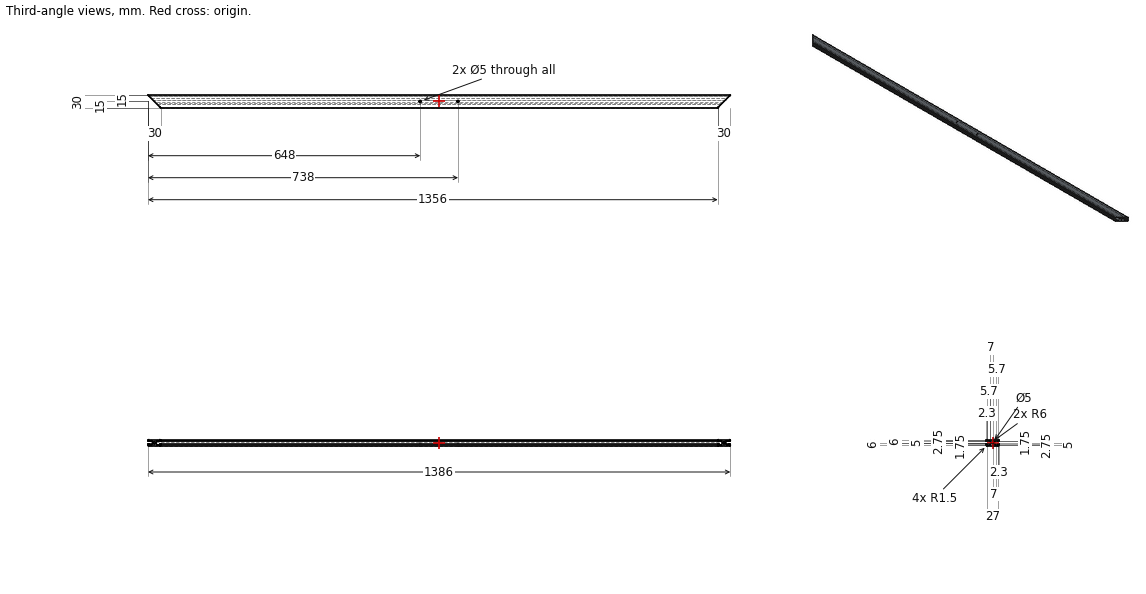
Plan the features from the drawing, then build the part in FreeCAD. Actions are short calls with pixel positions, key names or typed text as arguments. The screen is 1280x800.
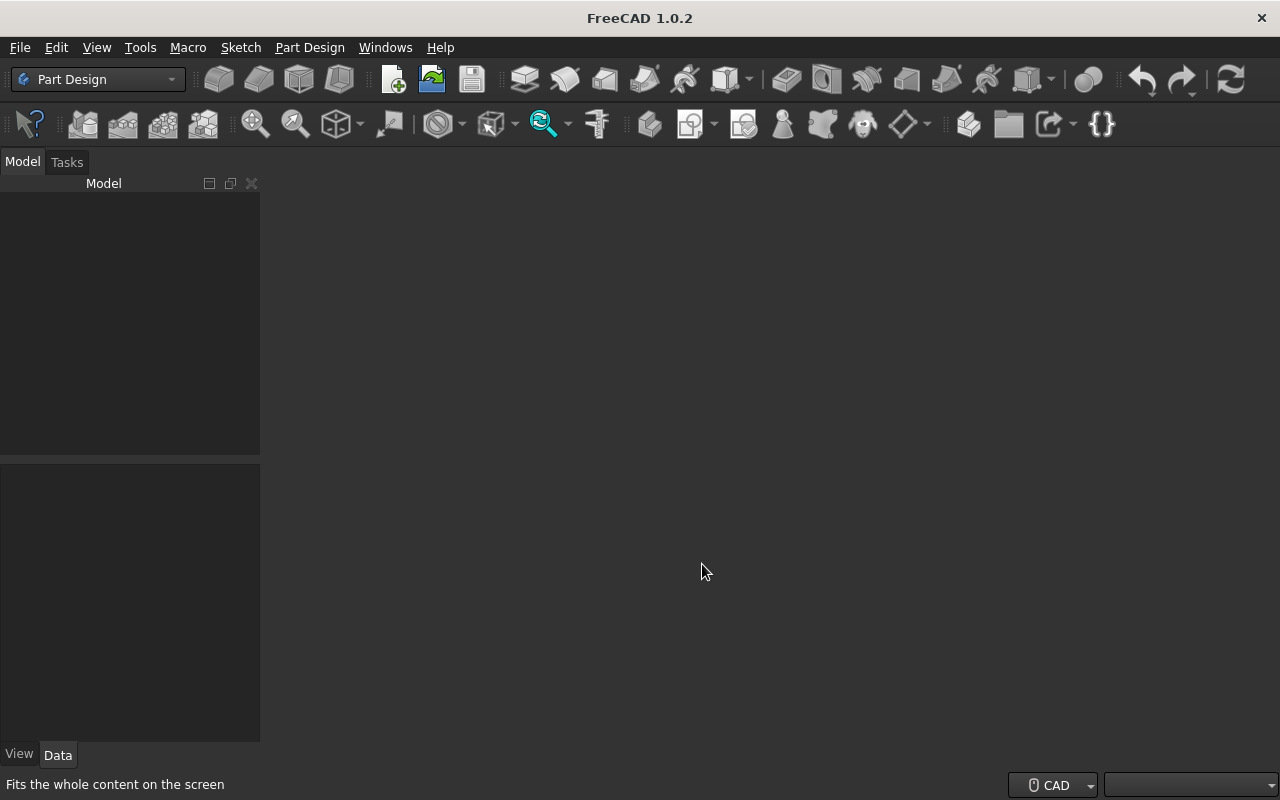
click(392, 80)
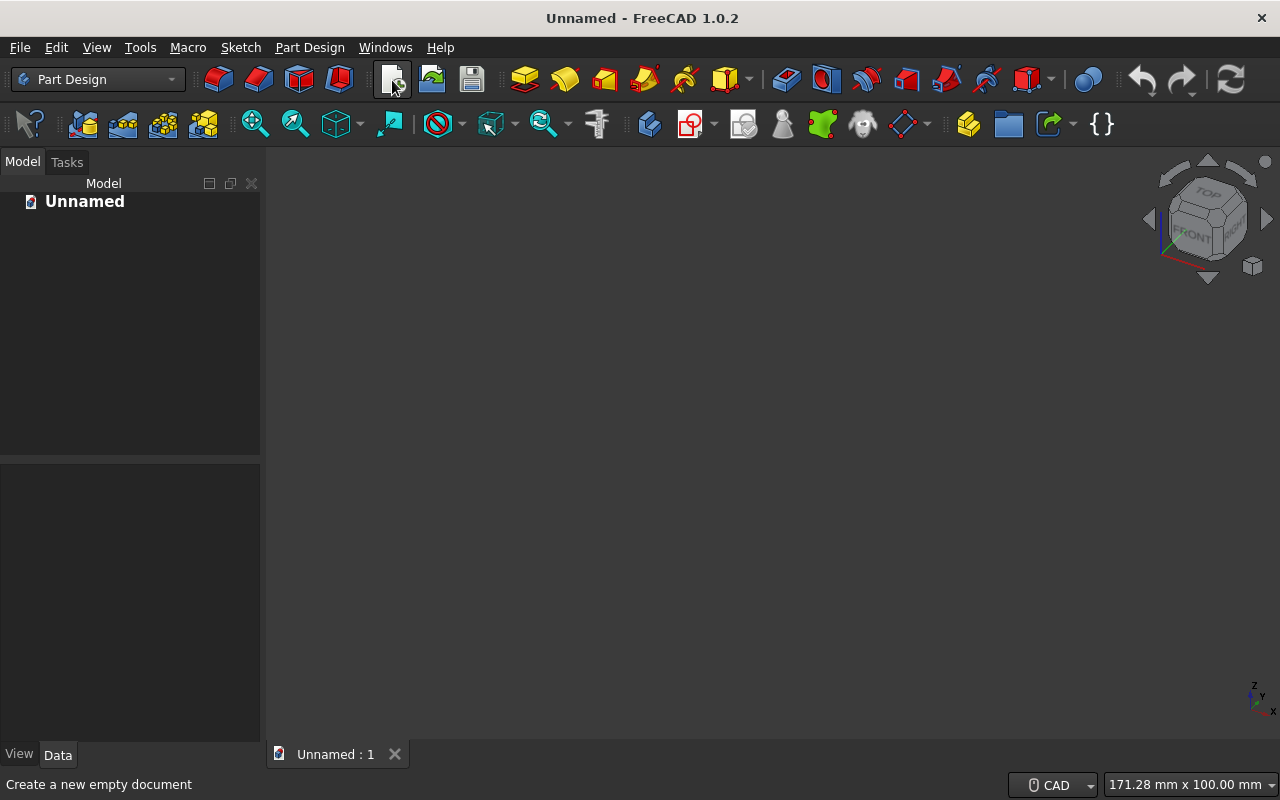
click(650, 124)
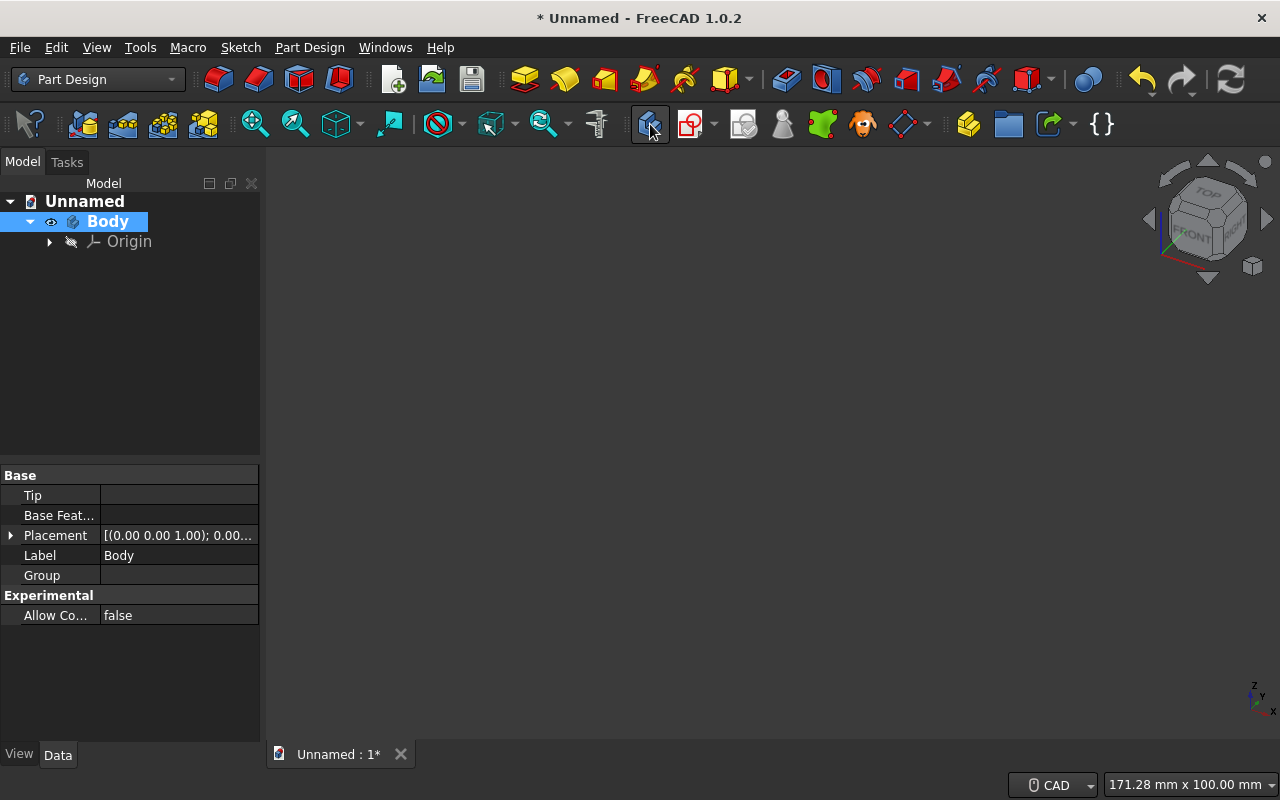
click(50, 242)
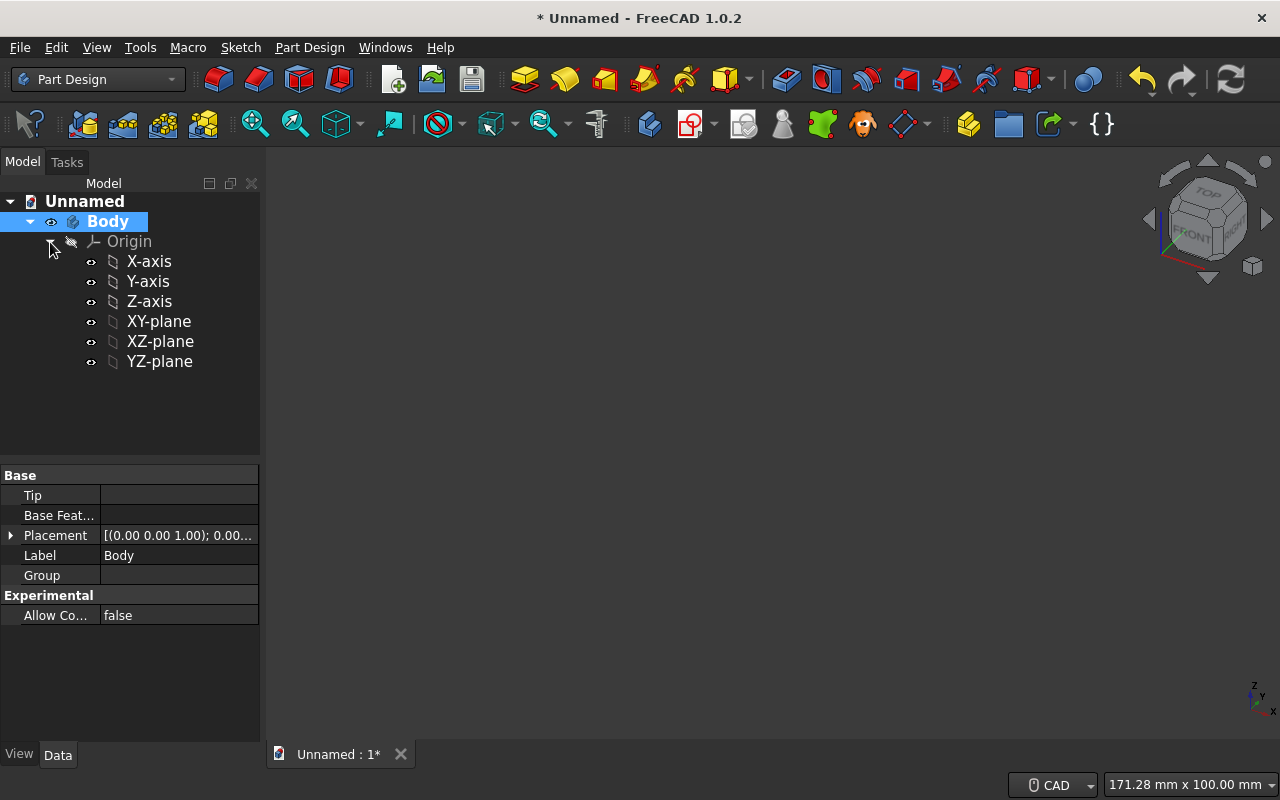
click(136, 362)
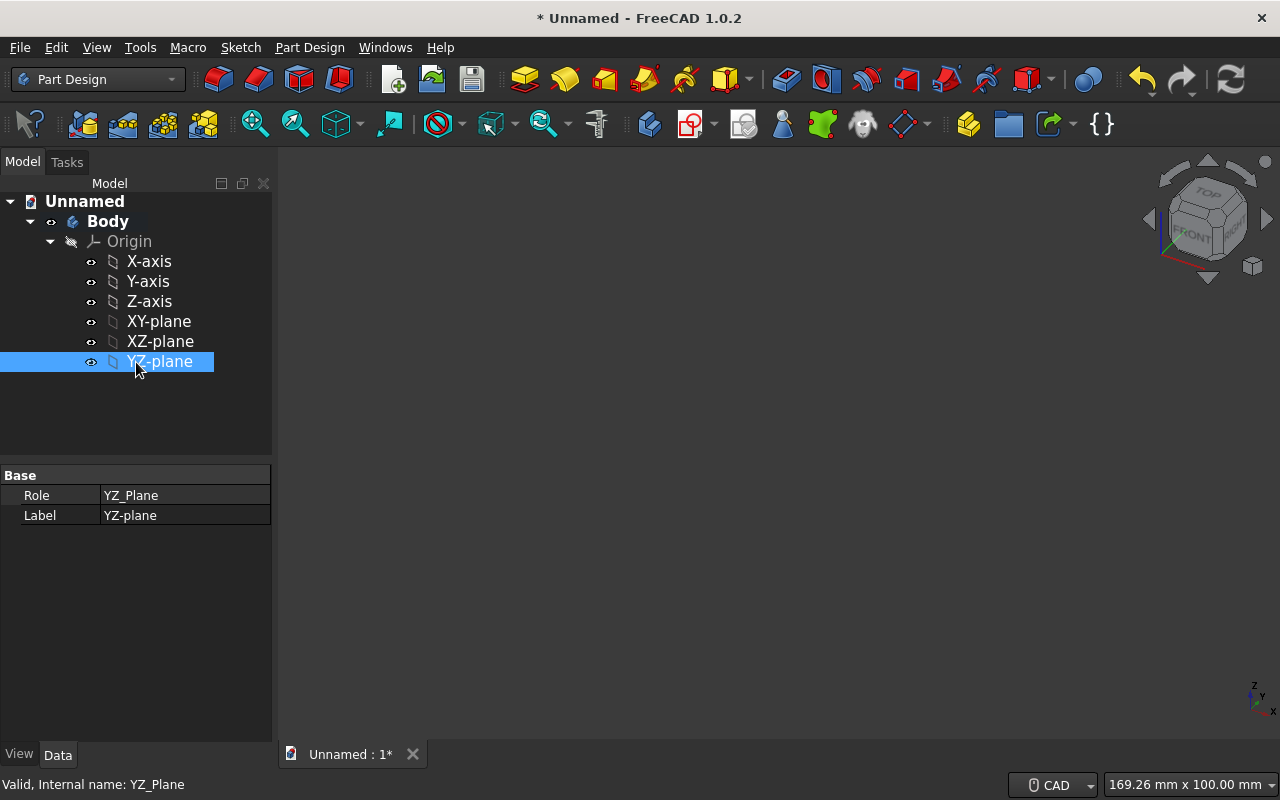
click(904, 124)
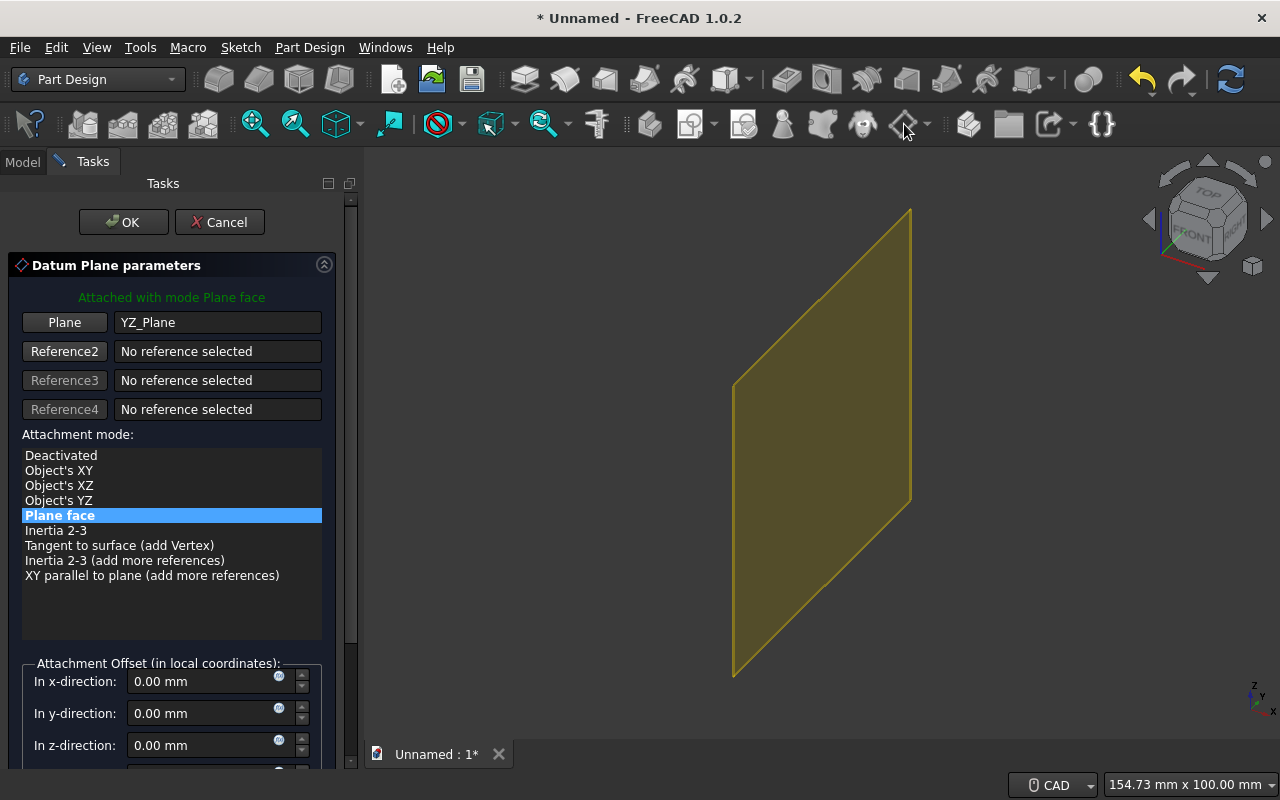
triple_click(210, 745)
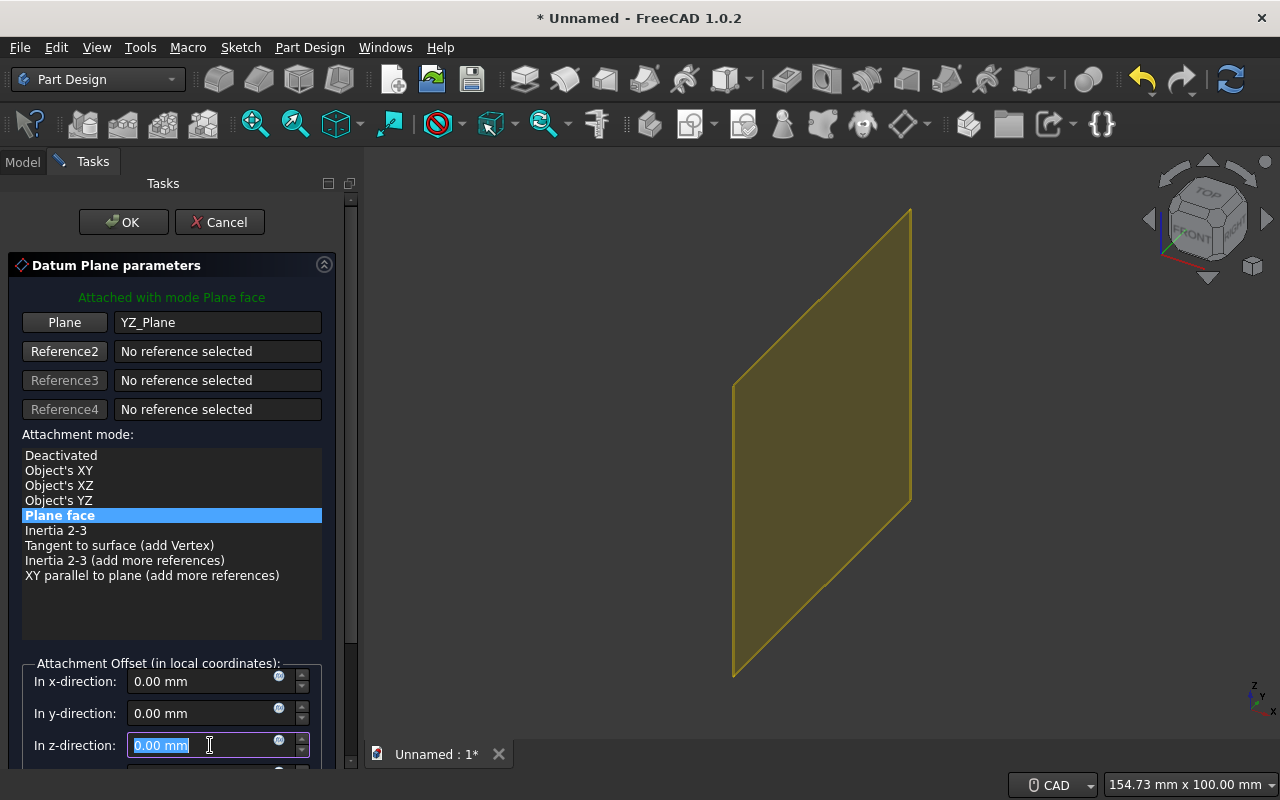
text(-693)
key(Tab)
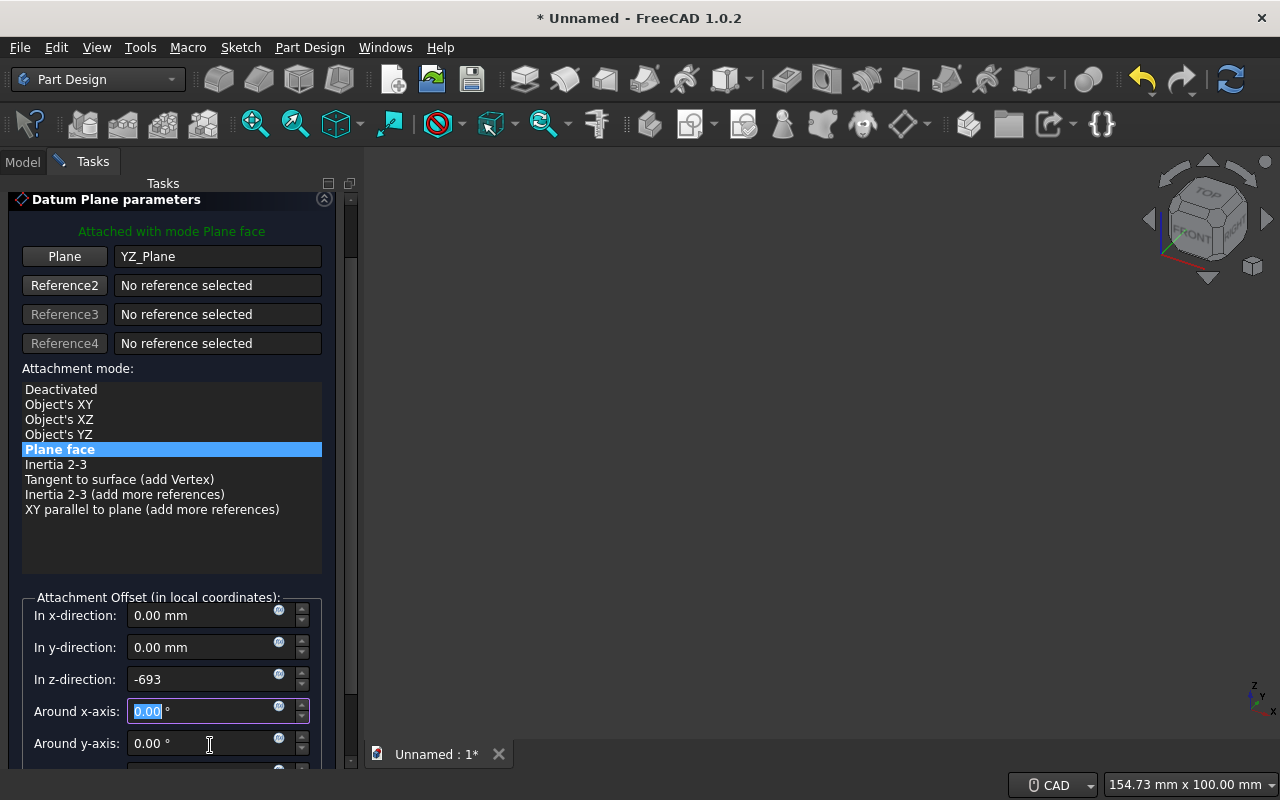
scroll(351, 480, up, 2)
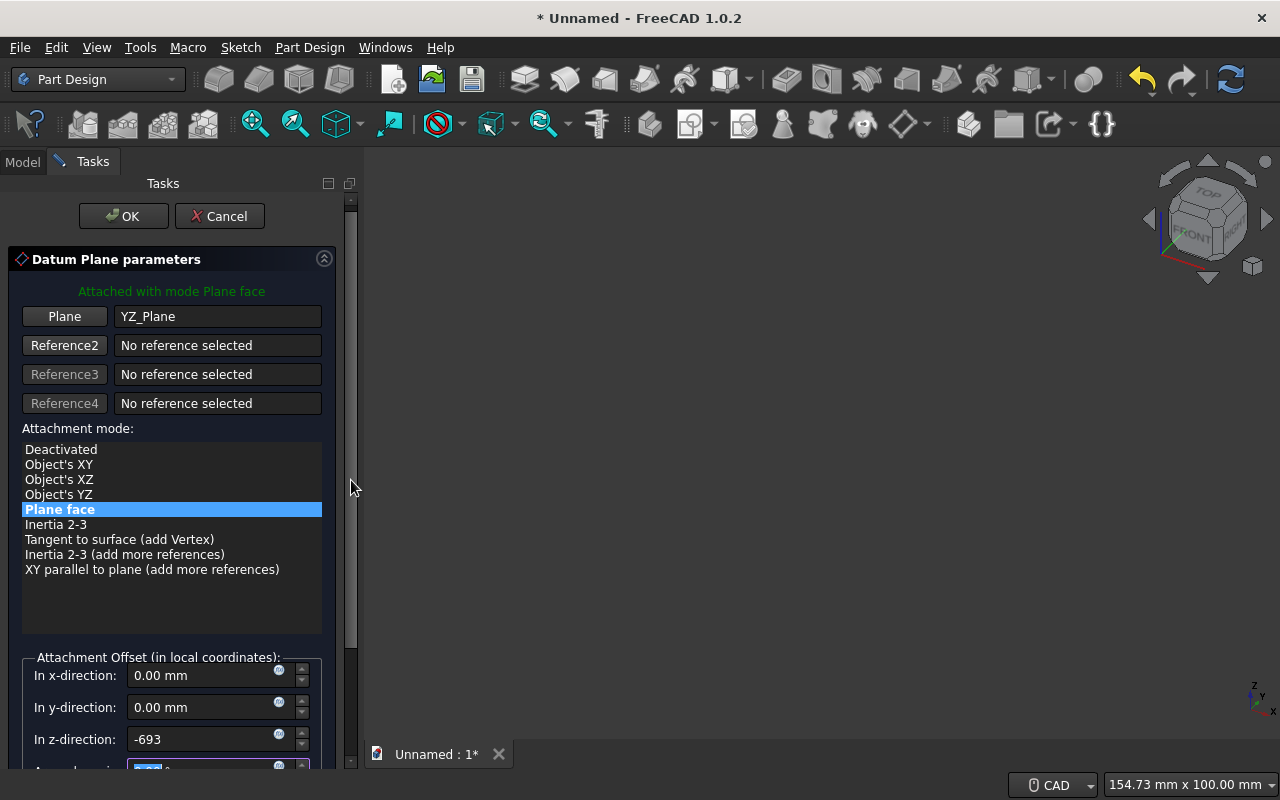
click(124, 222)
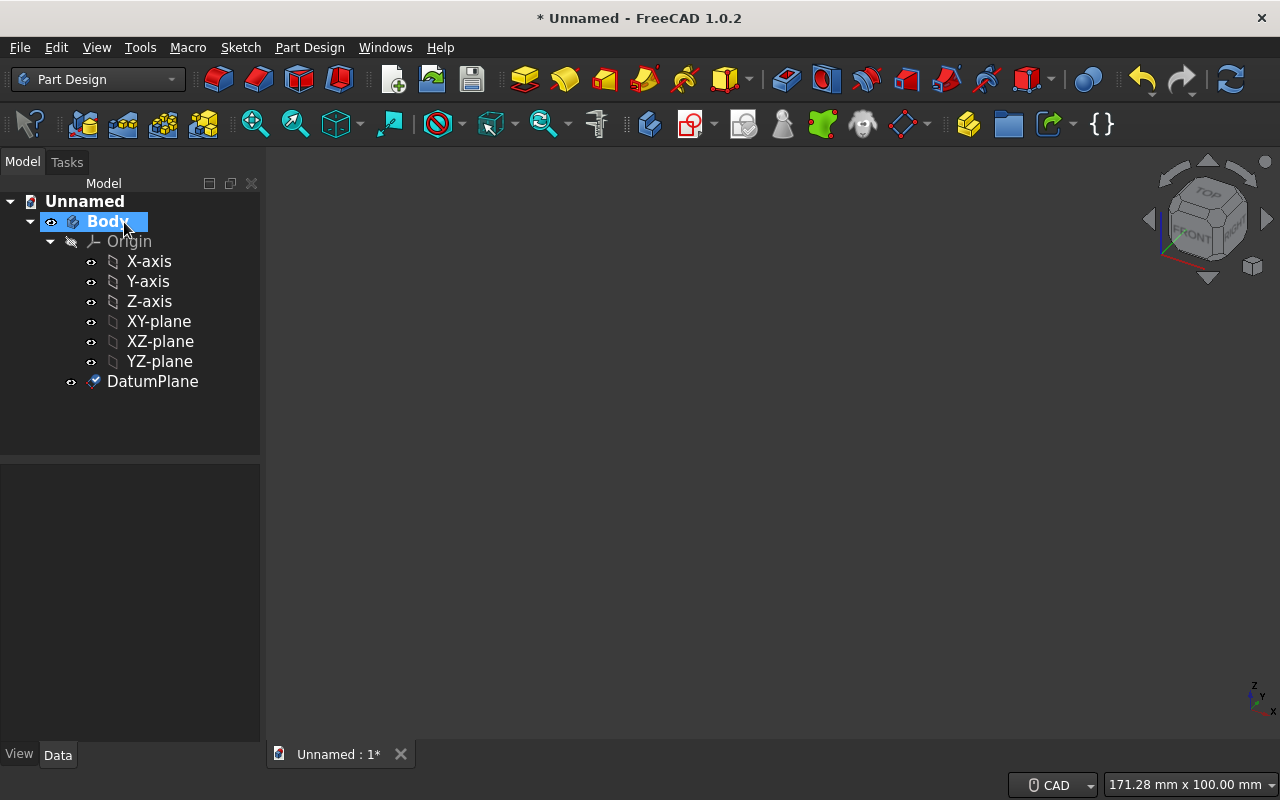
click(116, 382)